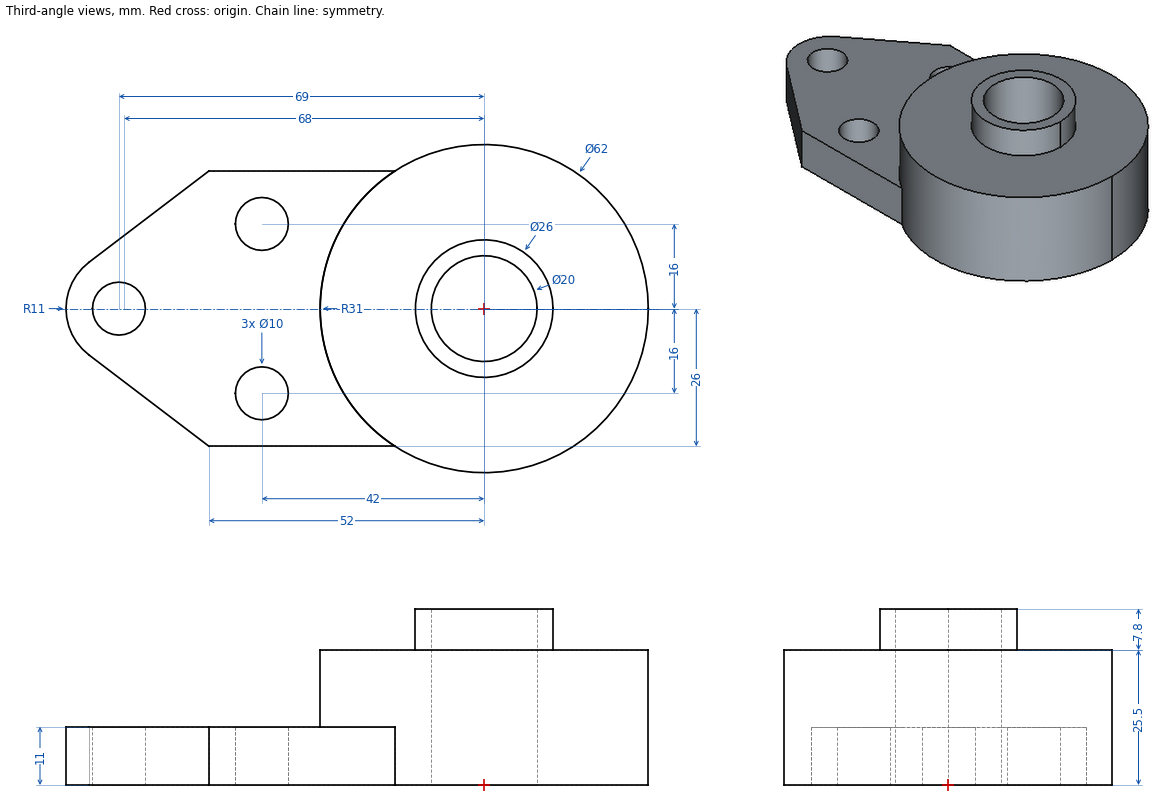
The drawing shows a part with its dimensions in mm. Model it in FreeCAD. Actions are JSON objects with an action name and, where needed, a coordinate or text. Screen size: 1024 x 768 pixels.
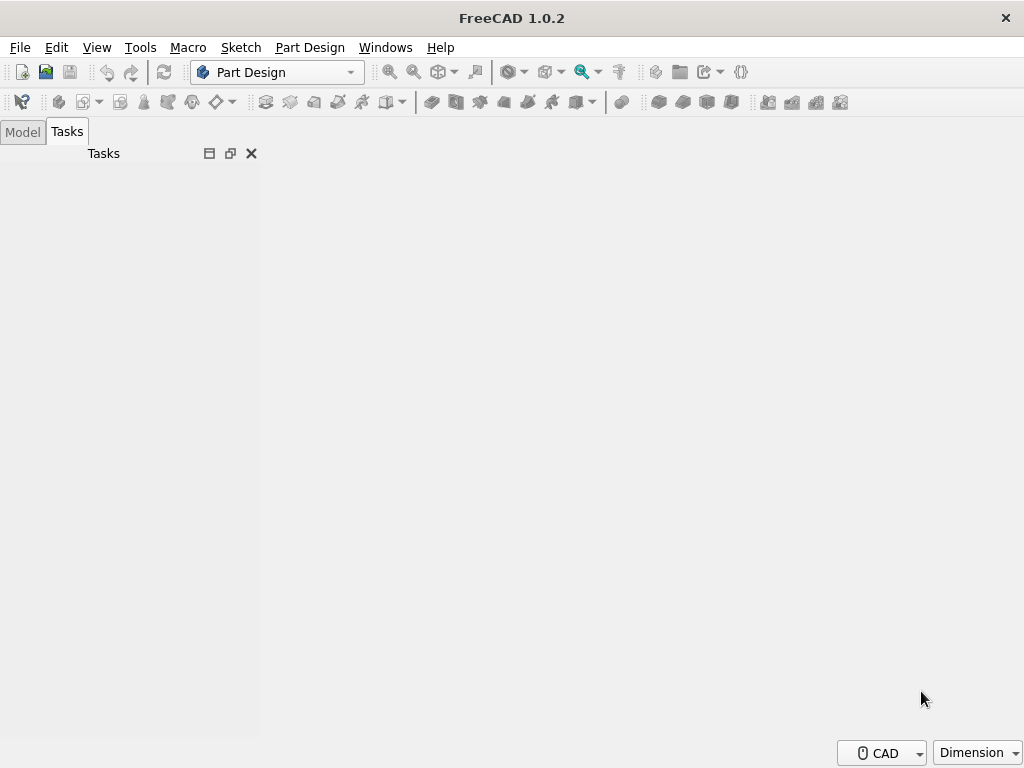
{"action": "left_click", "coordinate": [22, 72]}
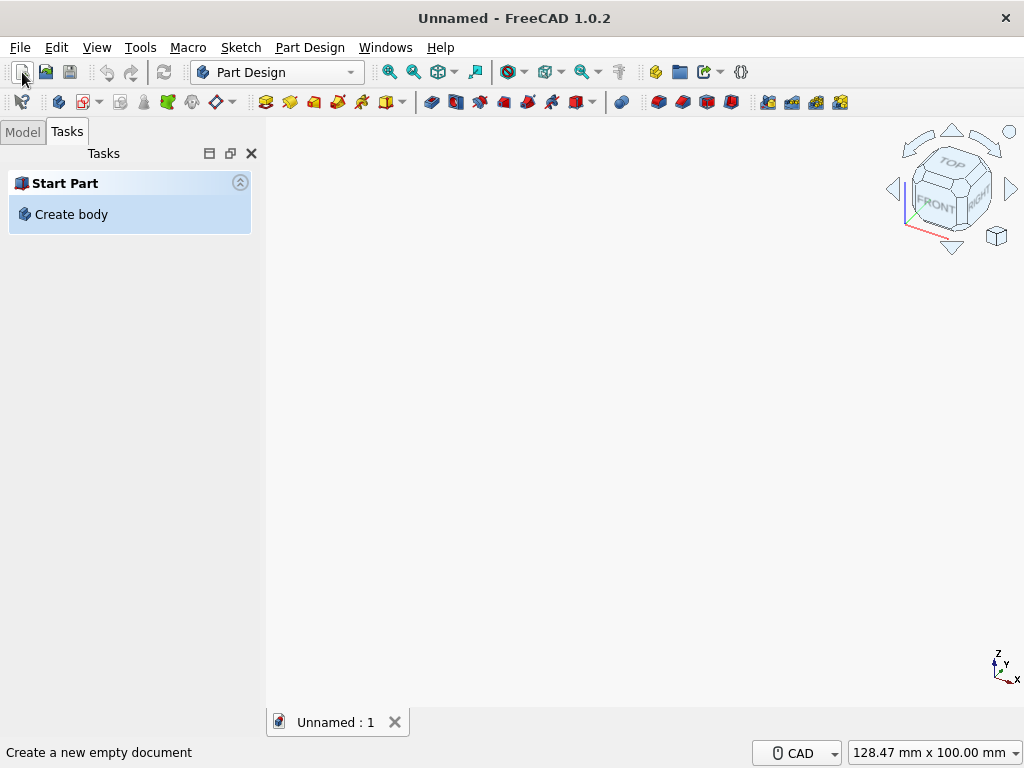
{"action": "left_click", "coordinate": [84, 102]}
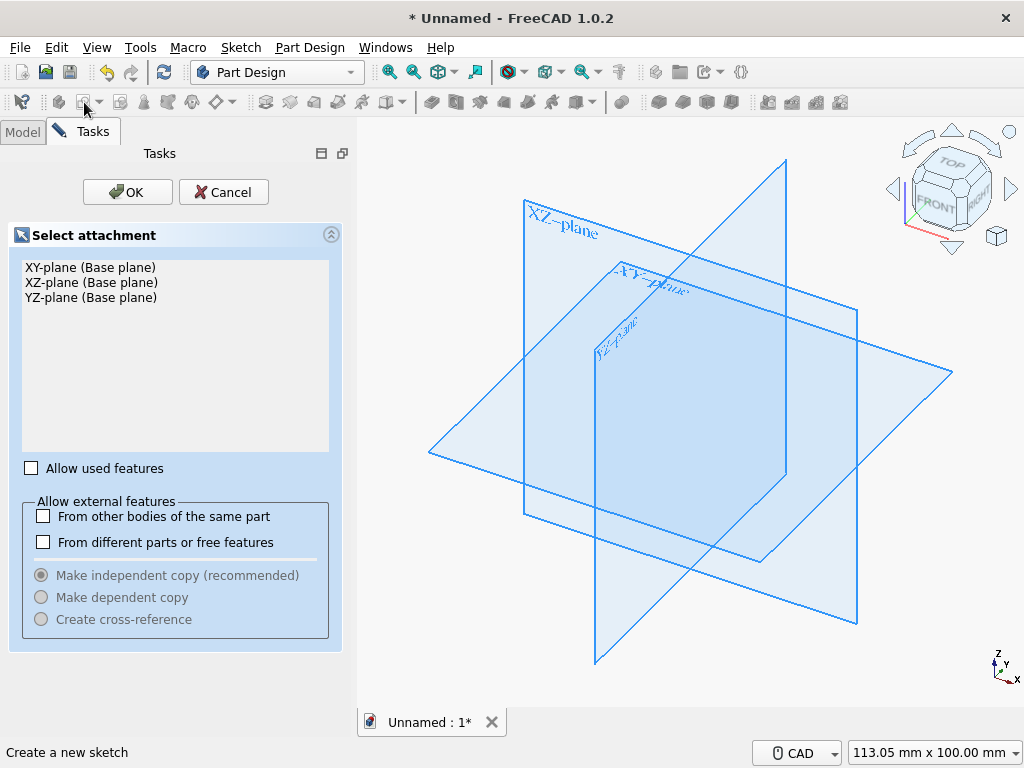
{"action": "left_click", "coordinate": [82, 268]}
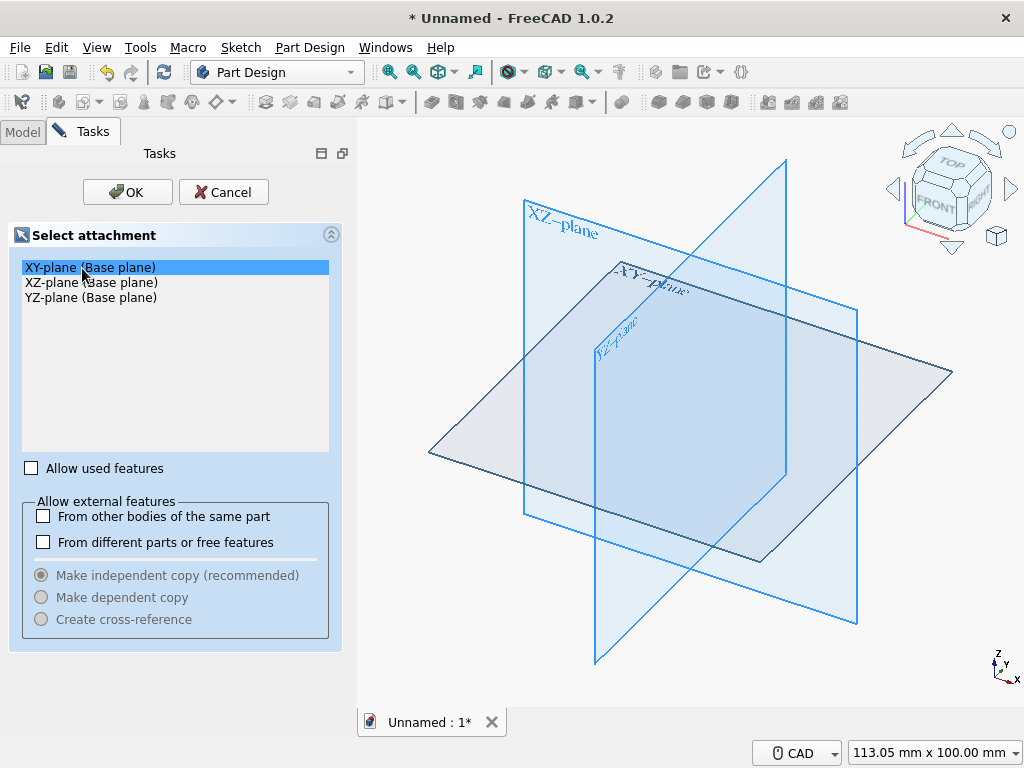
{"action": "left_click", "coordinate": [128, 192]}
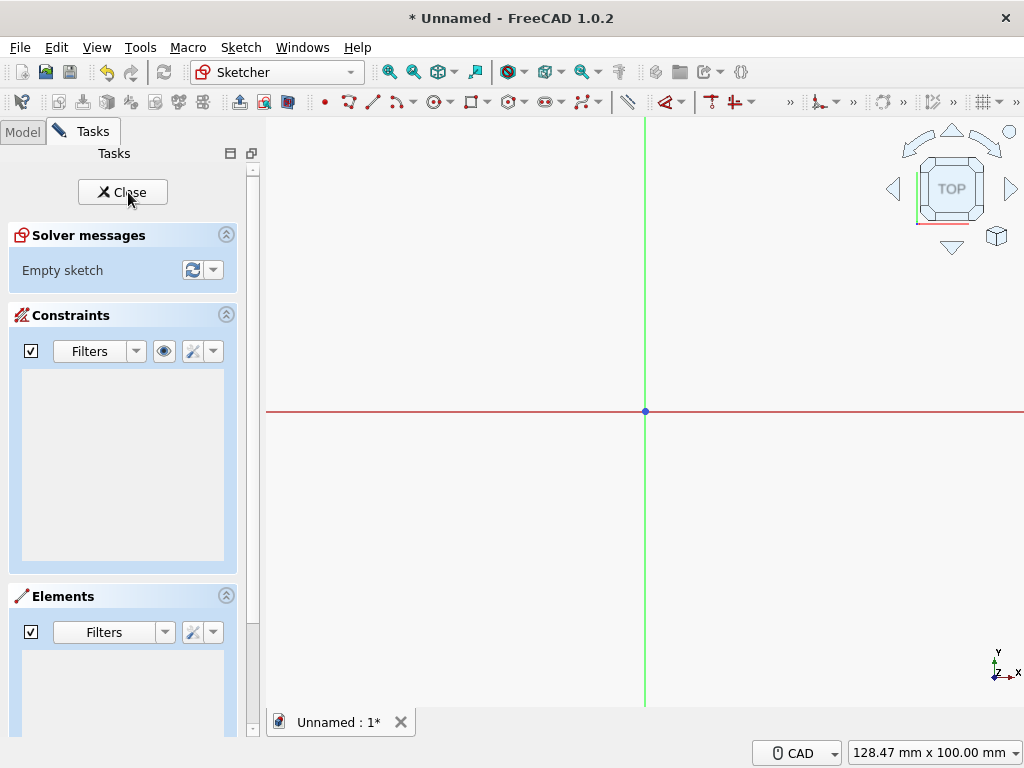
{"action": "left_click", "coordinate": [434, 102]}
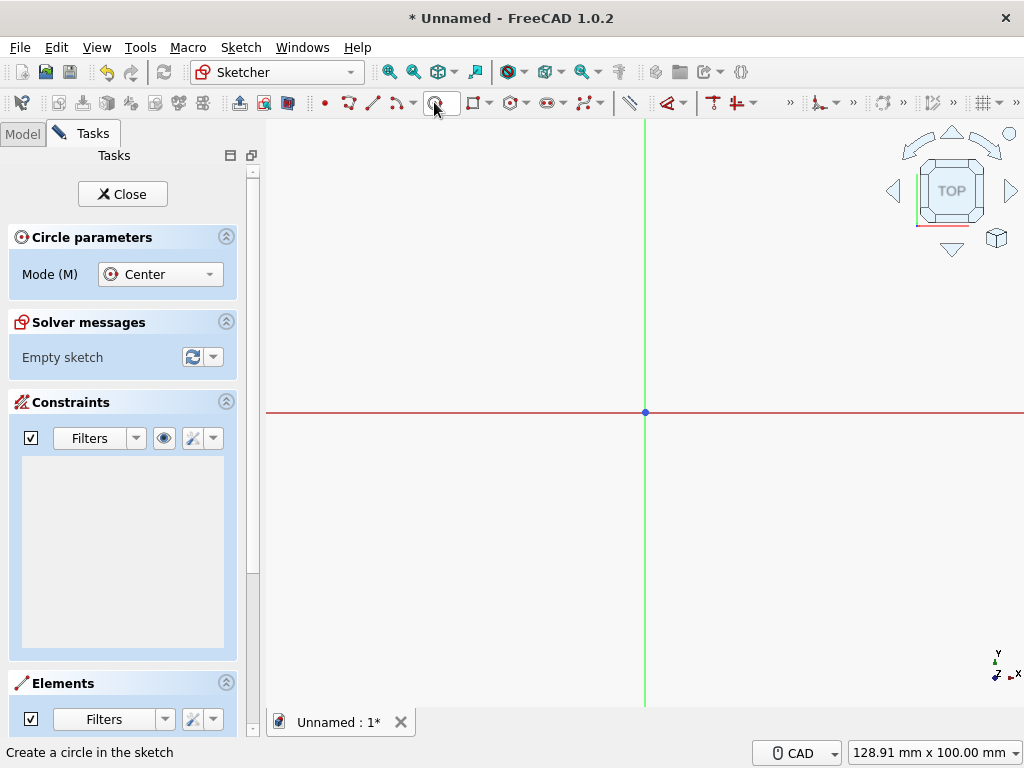
{"action": "left_click", "coordinate": [645, 413]}
{"action": "mouse_move", "coordinate": [774, 284]}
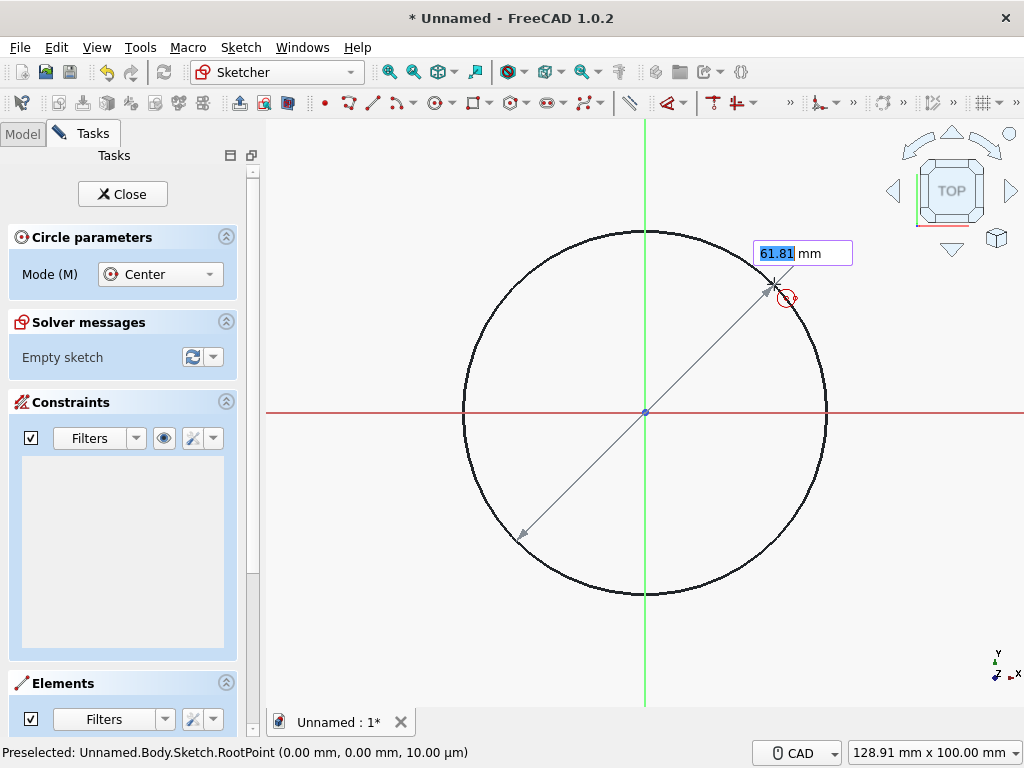
{"action": "type", "text": "62"}
{"action": "key", "text": "Return"}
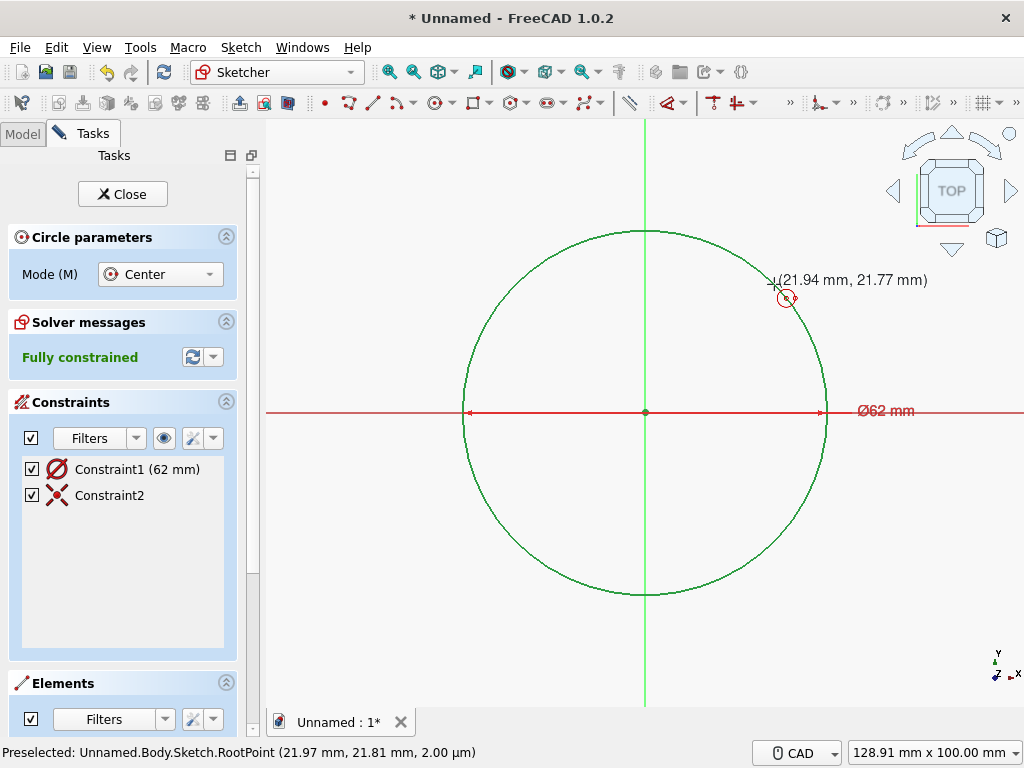
{"action": "left_click", "coordinate": [645, 413]}
{"action": "mouse_move", "coordinate": [687, 371]}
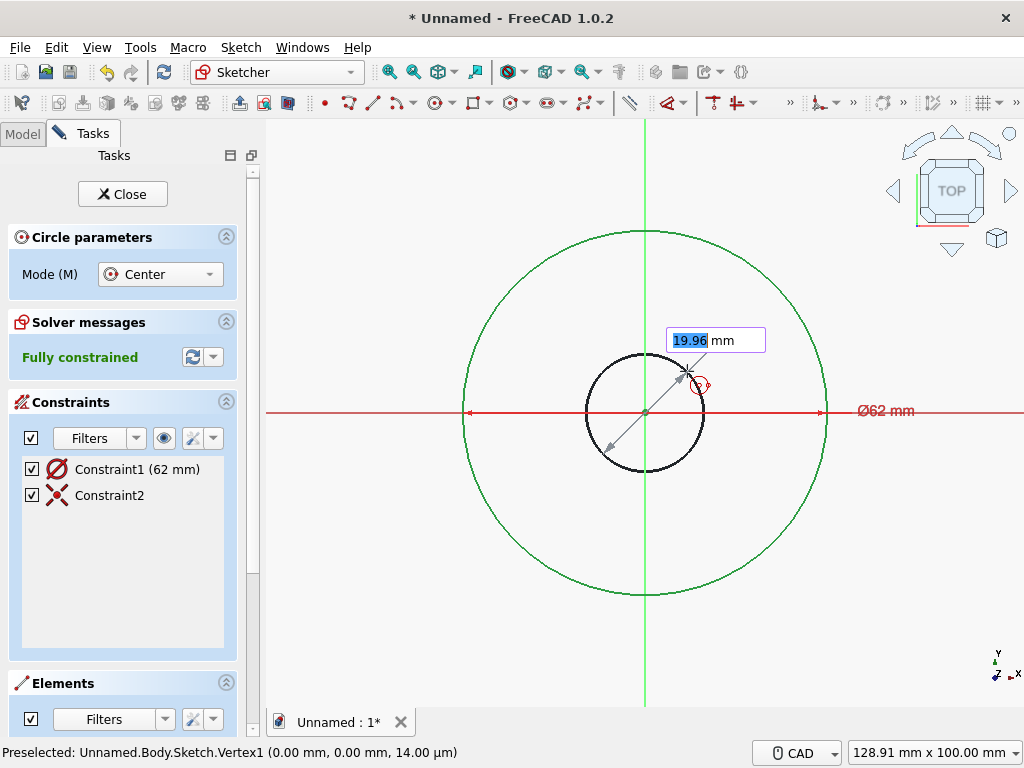
{"action": "type", "text": "20"}
{"action": "key", "text": "Return"}
{"action": "key", "text": "Escape"}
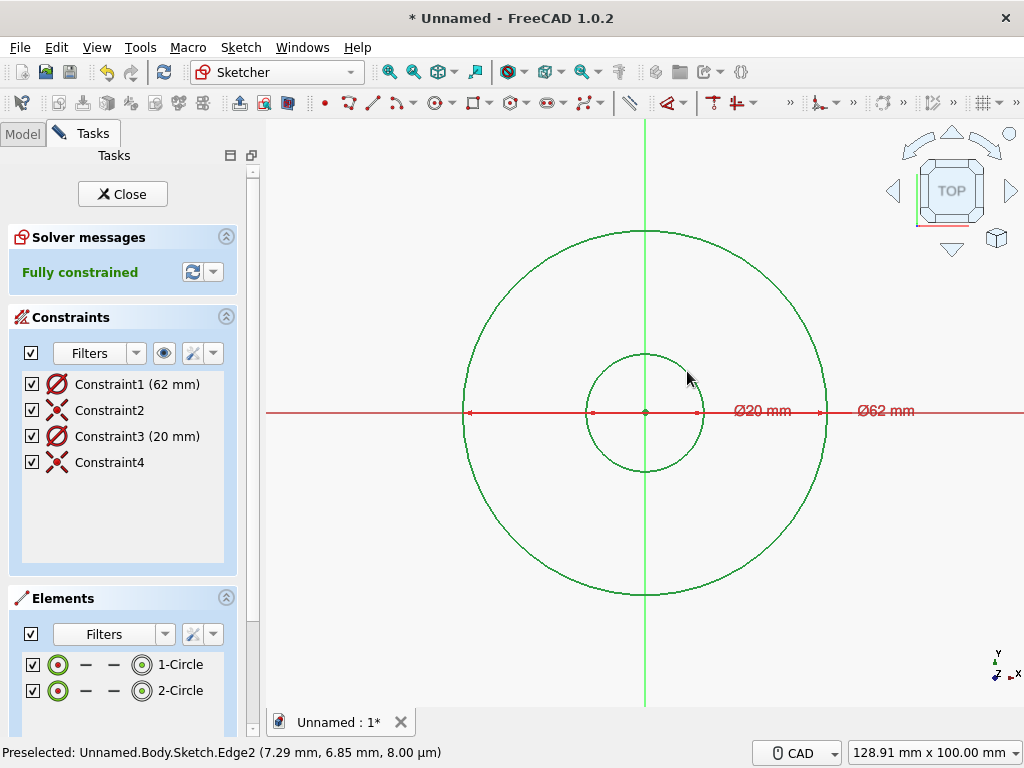
{"action": "left_click", "coordinate": [123, 194]}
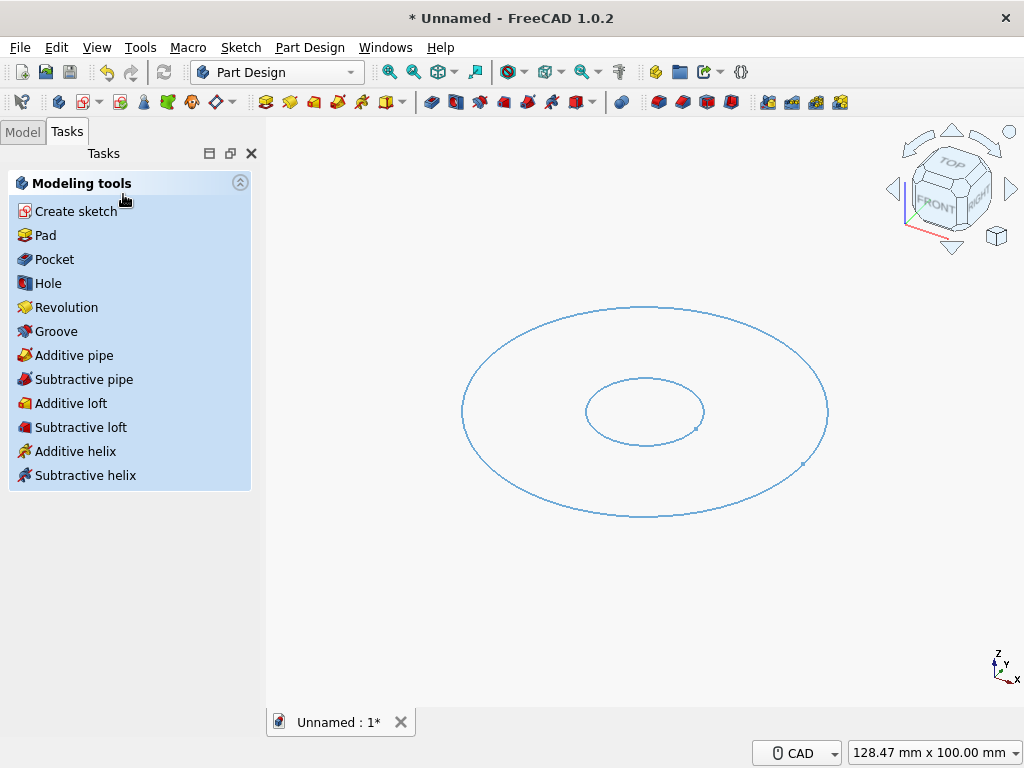
{"action": "left_click", "coordinate": [266, 102]}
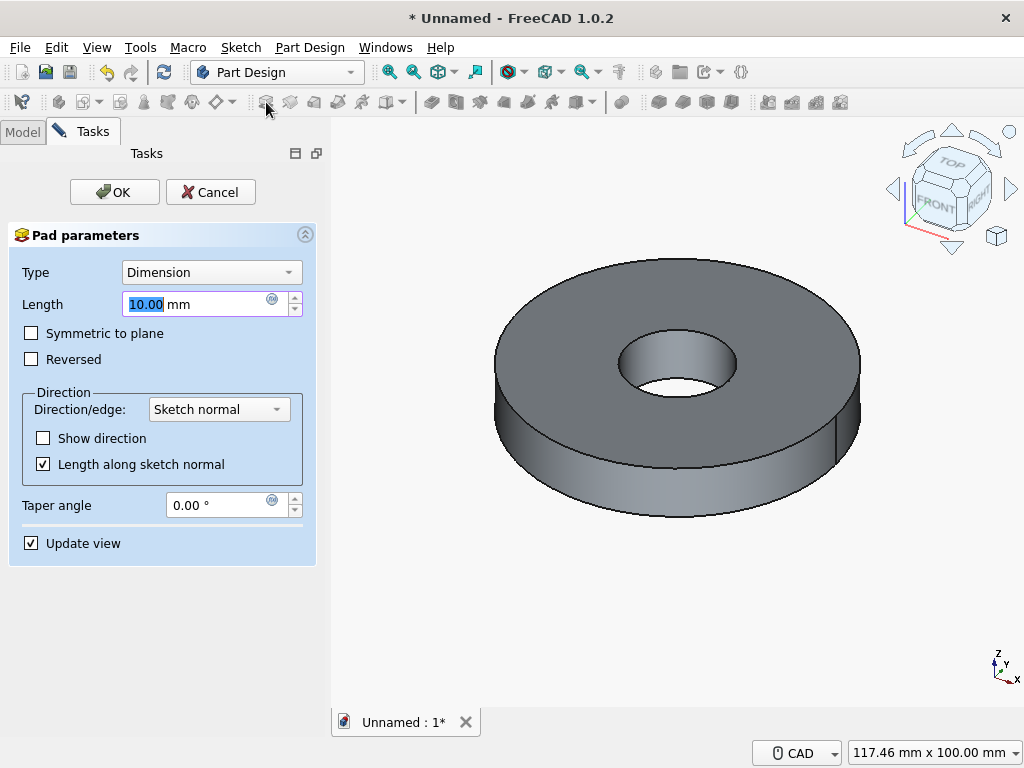
{"action": "type", "text": "25.5"}
{"action": "key", "text": "Tab"}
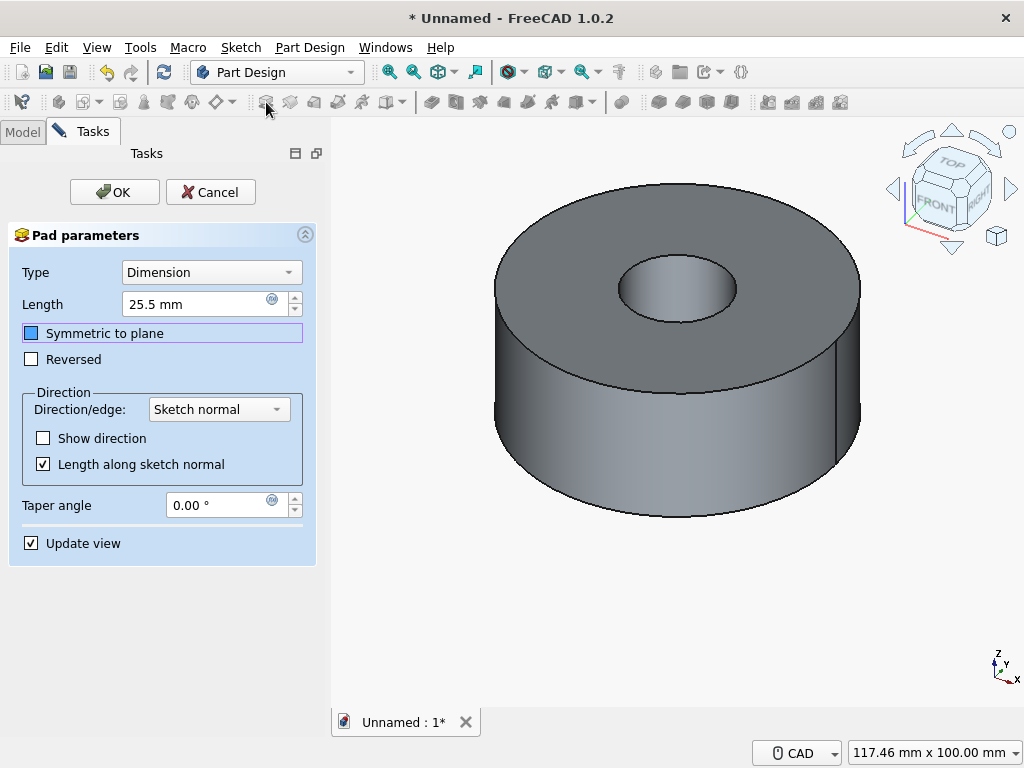
{"action": "left_click", "coordinate": [115, 192]}